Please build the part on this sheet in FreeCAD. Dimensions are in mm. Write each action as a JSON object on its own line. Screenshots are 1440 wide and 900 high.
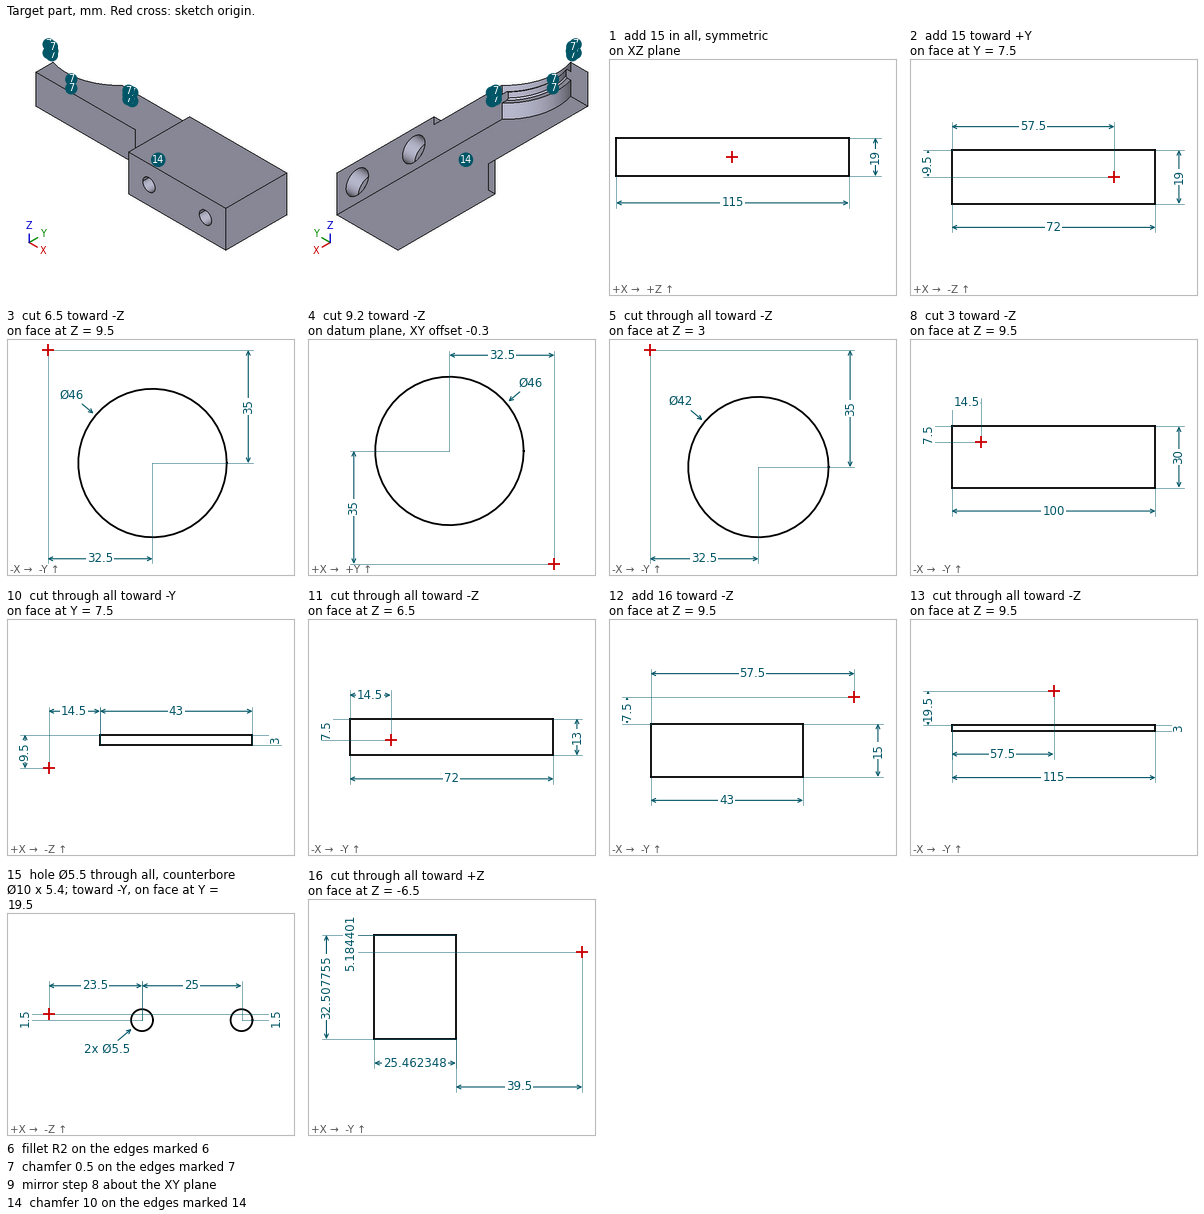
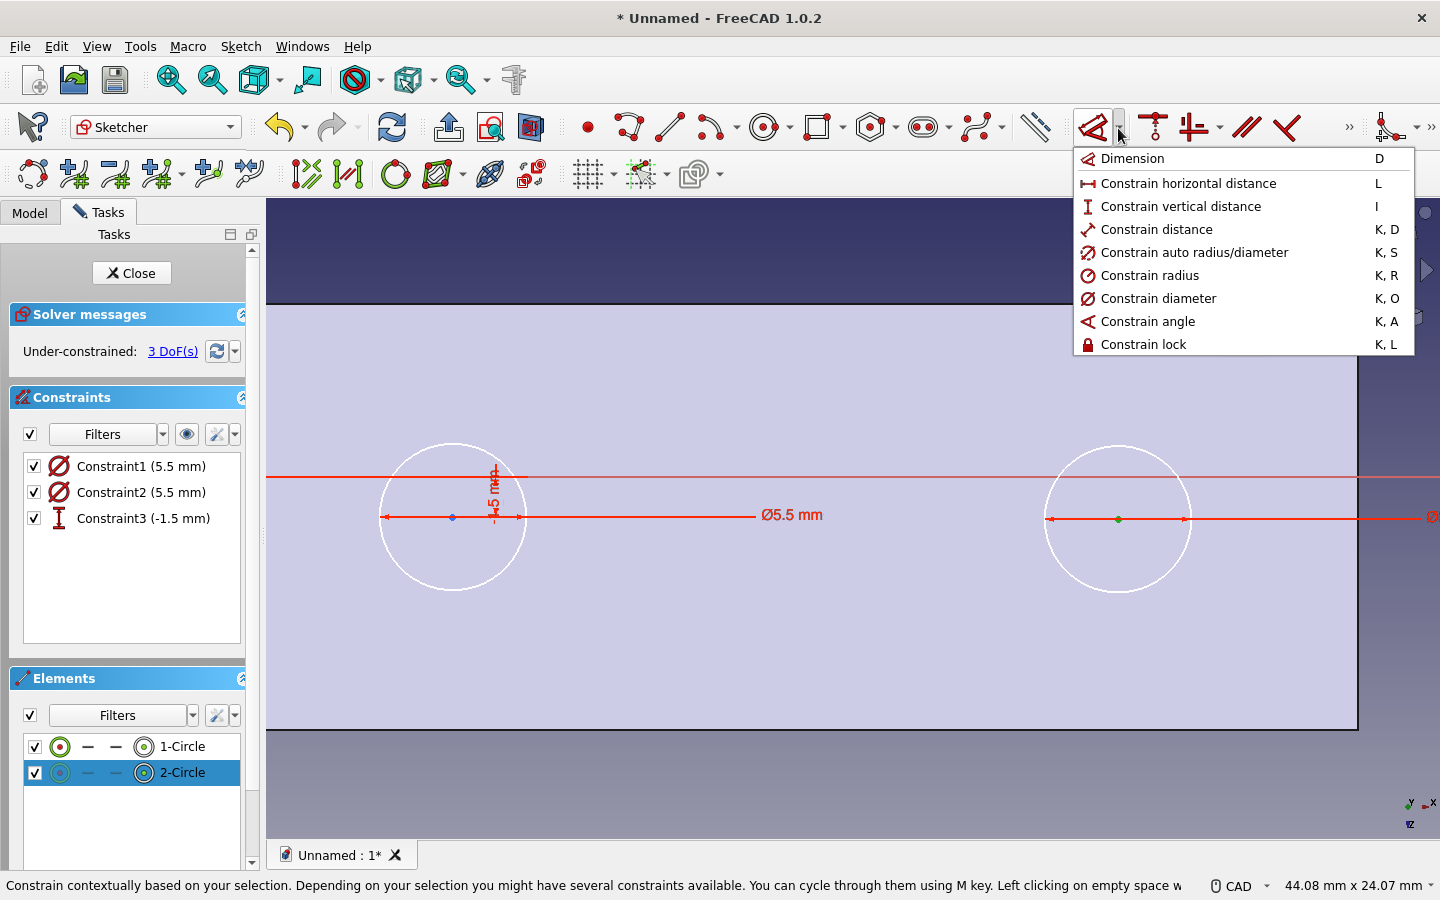
{"action": "left_click", "coordinate": [1244, 206]}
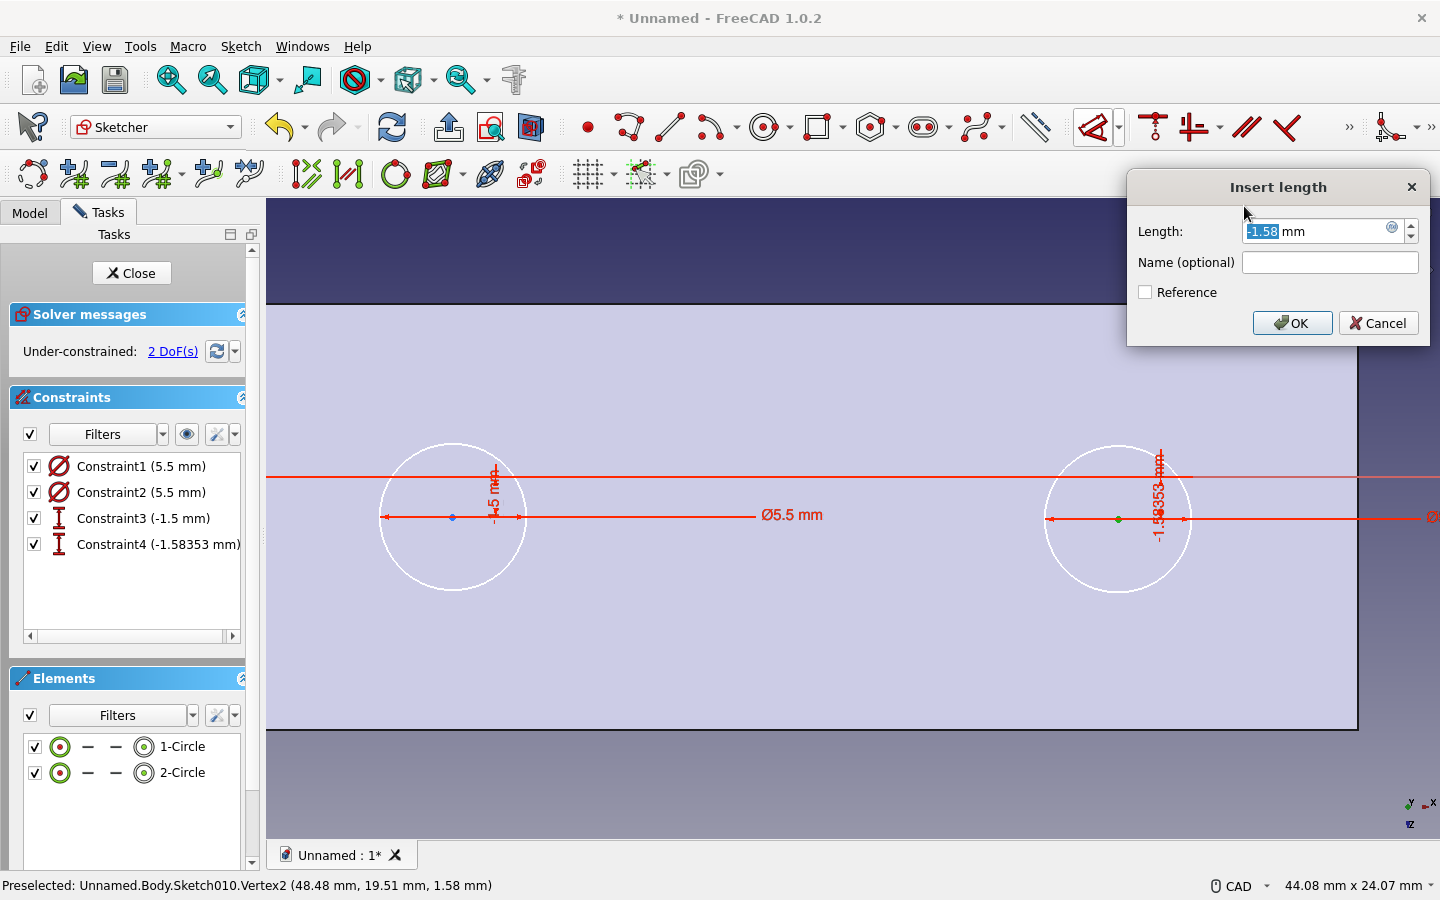
{"action": "type", "text": "-1.5"}
{"action": "key", "text": "Return"}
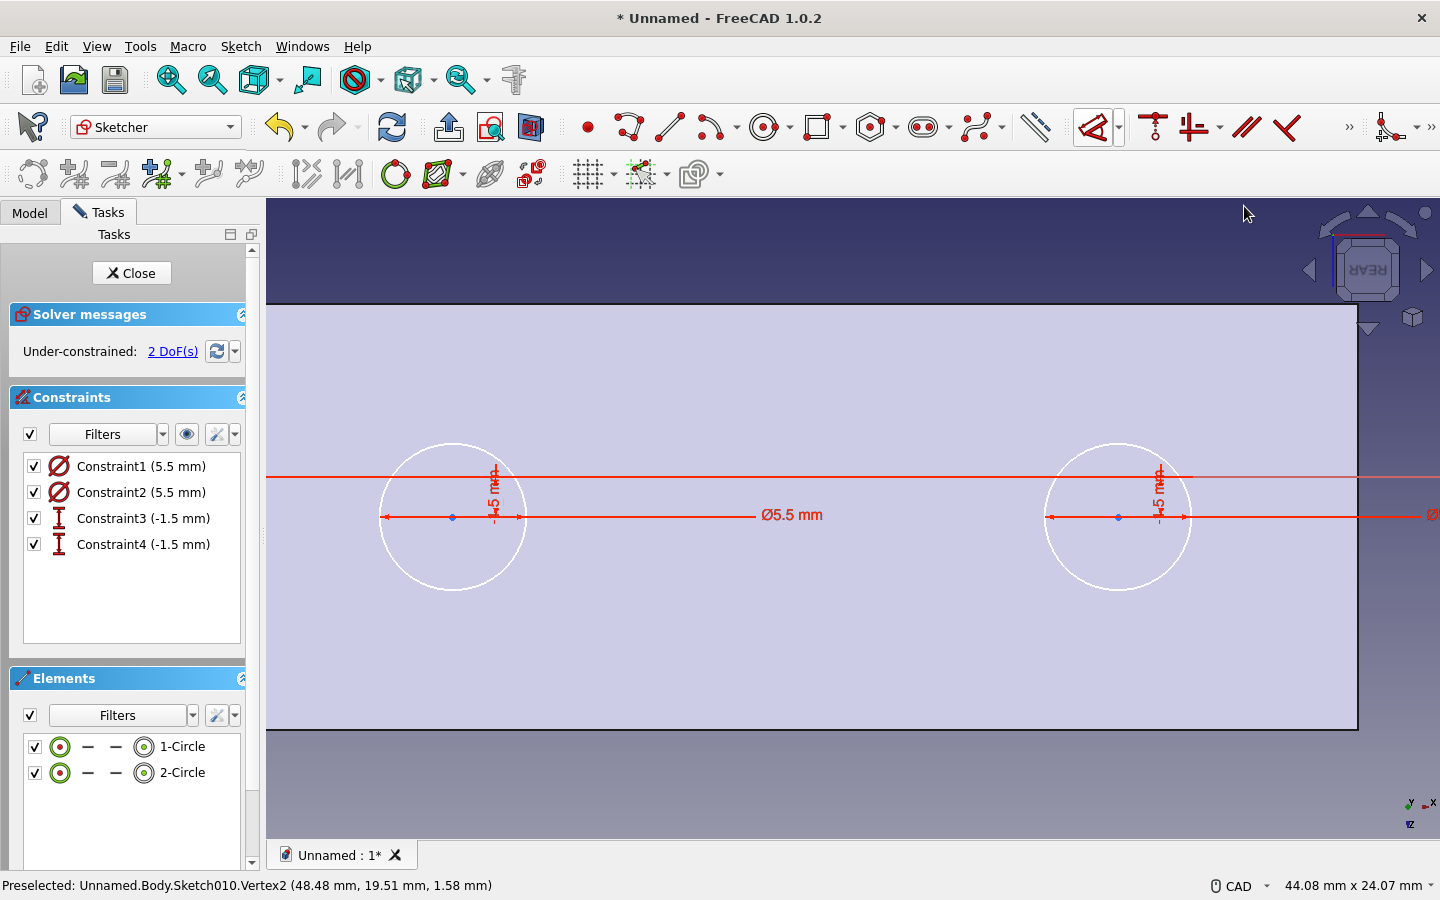
{"action": "left_click", "coordinate": [453, 517]}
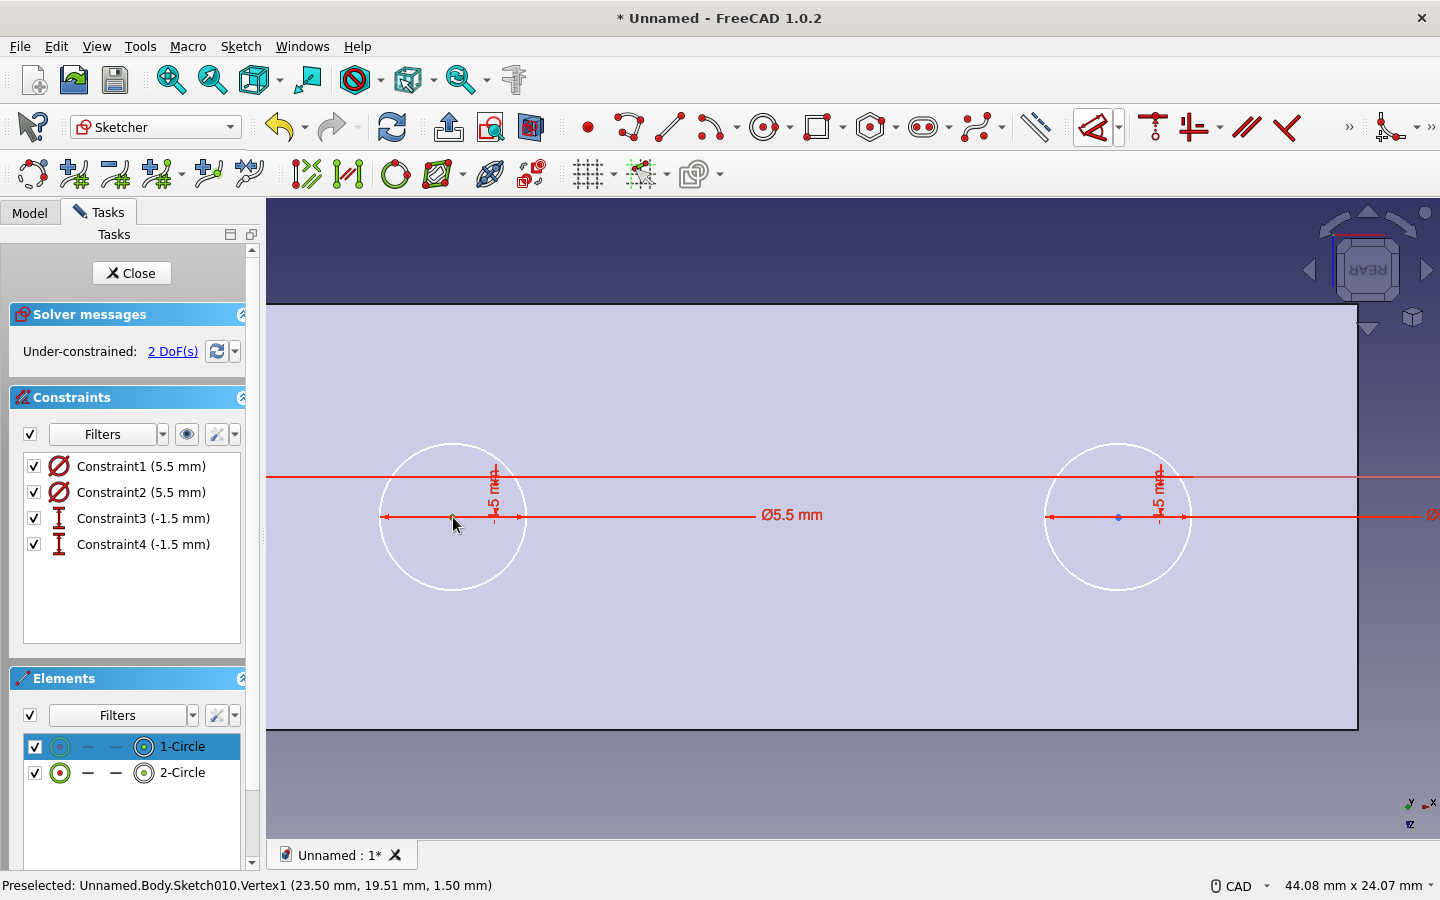
{"action": "left_click", "coordinate": [1118, 517]}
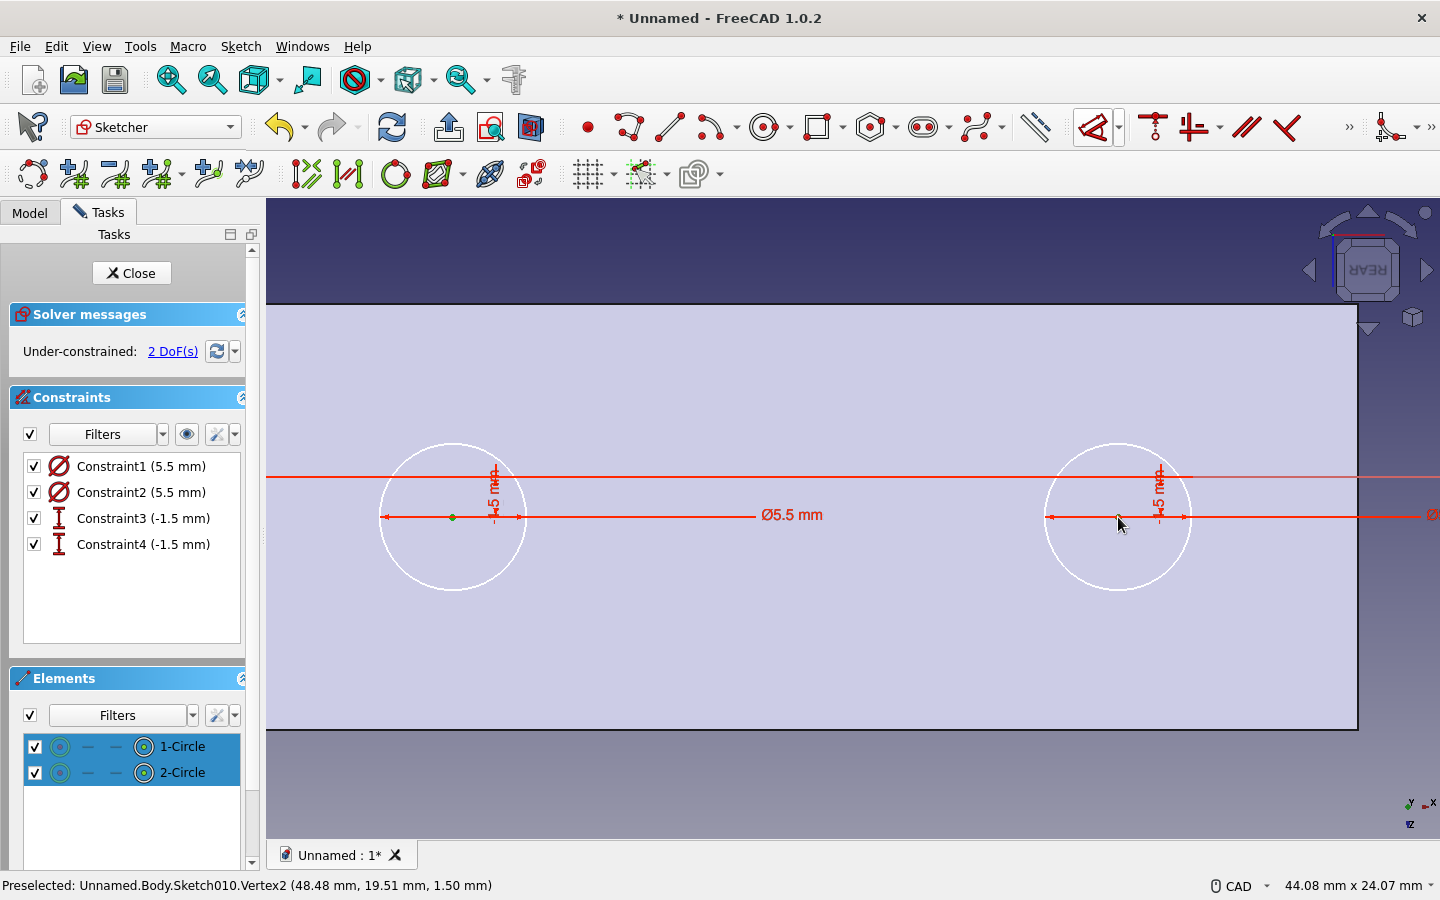
{"action": "left_click", "coordinate": [1118, 128]}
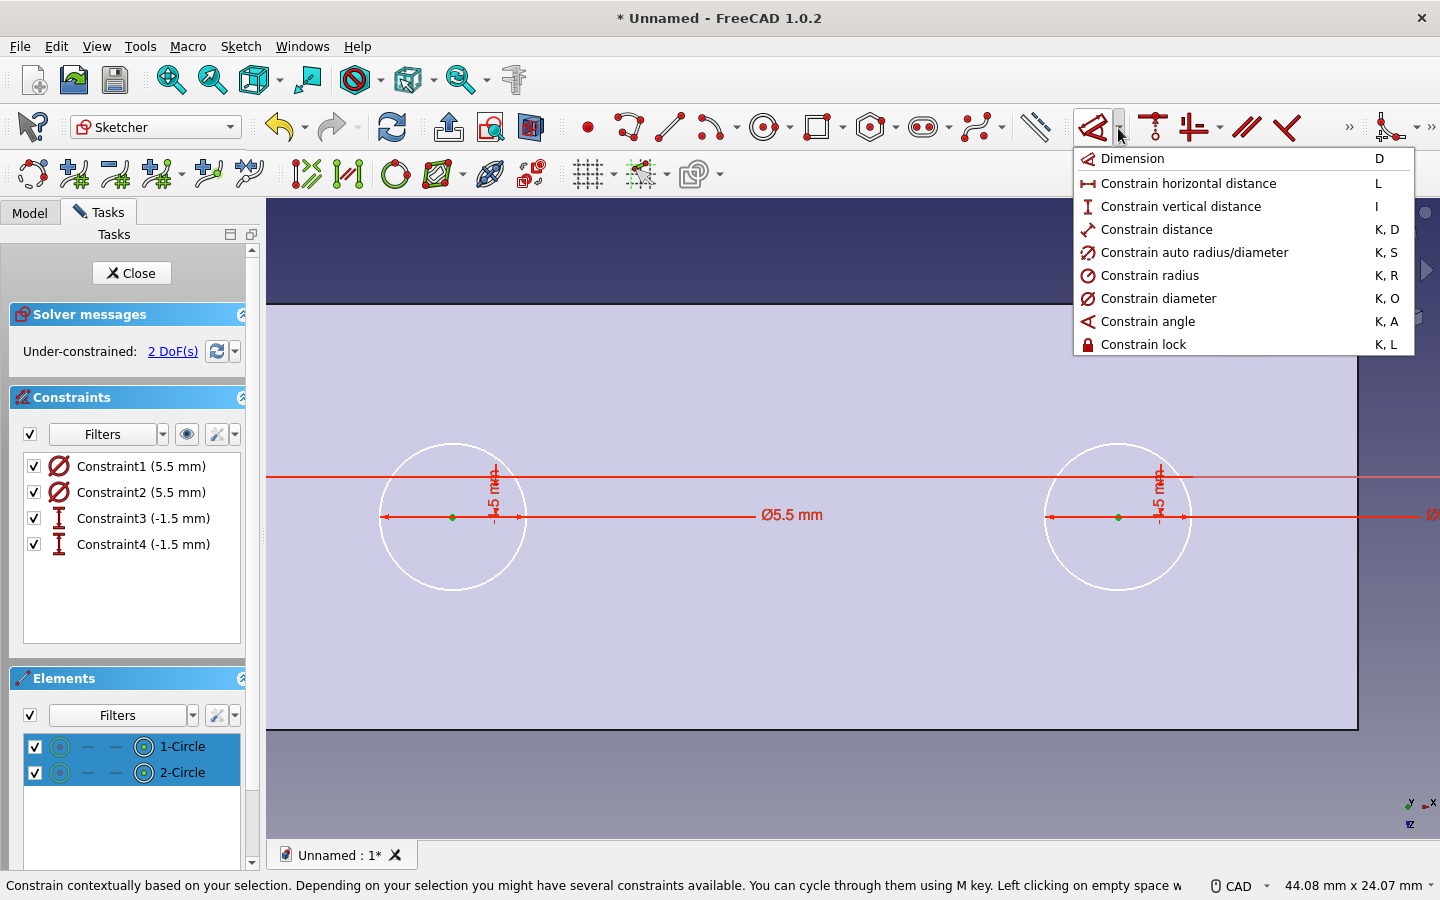
{"action": "left_click", "coordinate": [1244, 184]}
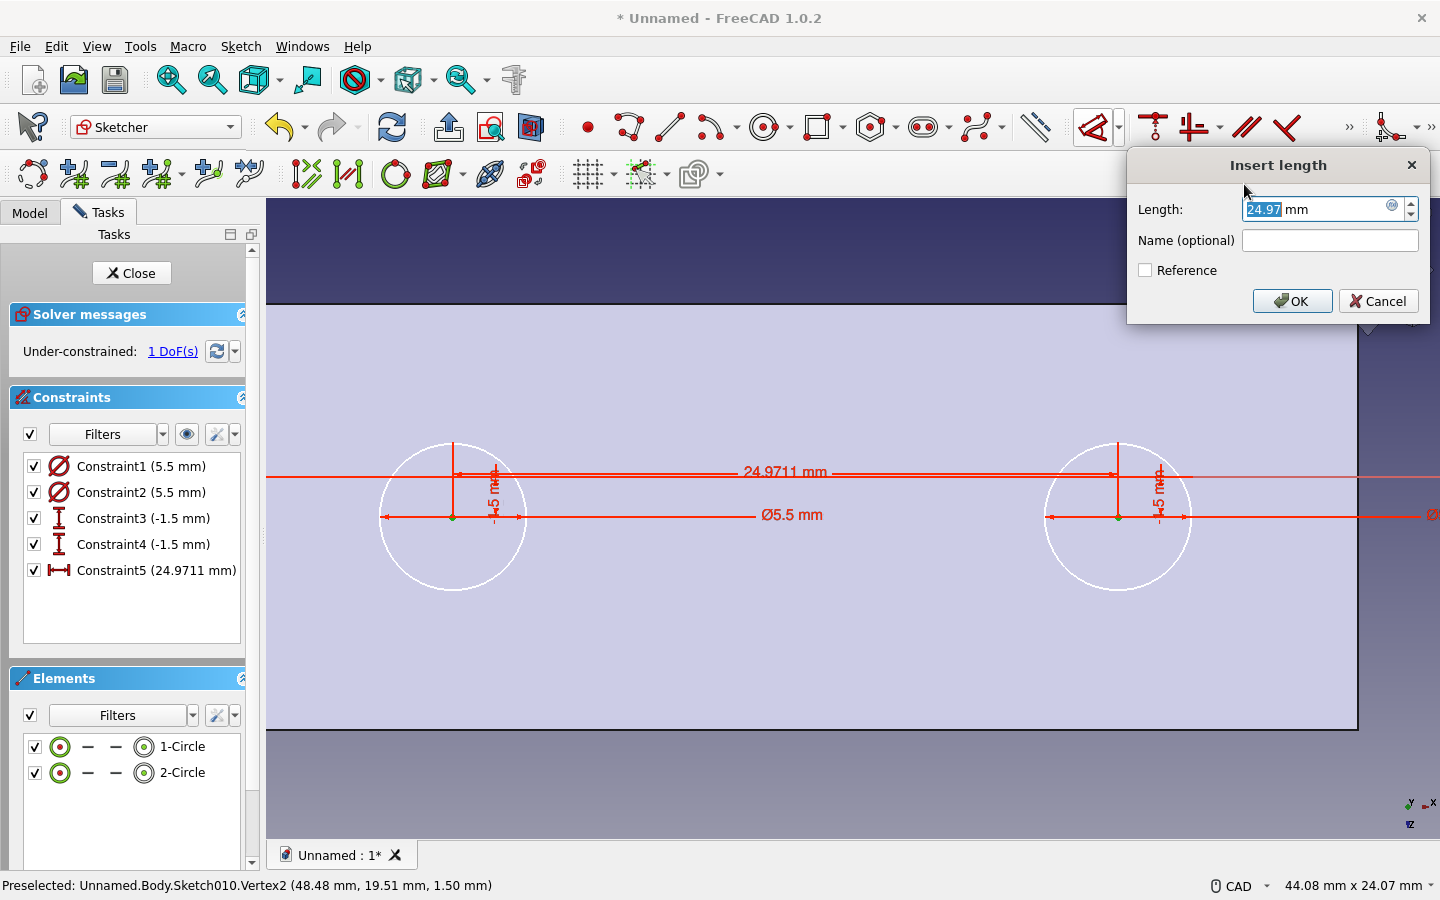
{"action": "type", "text": "25"}
{"action": "key", "text": "Return"}